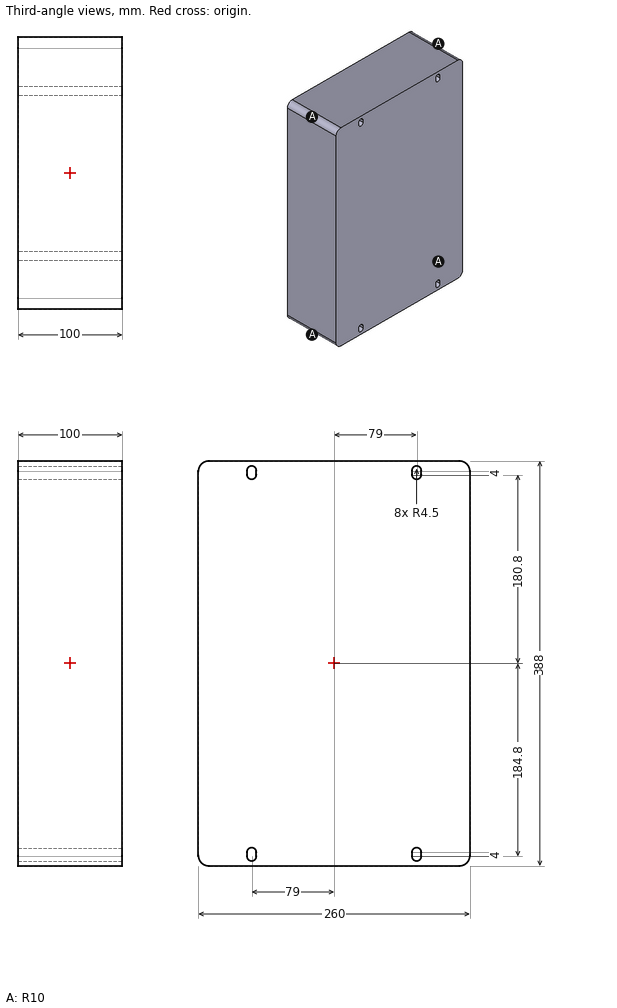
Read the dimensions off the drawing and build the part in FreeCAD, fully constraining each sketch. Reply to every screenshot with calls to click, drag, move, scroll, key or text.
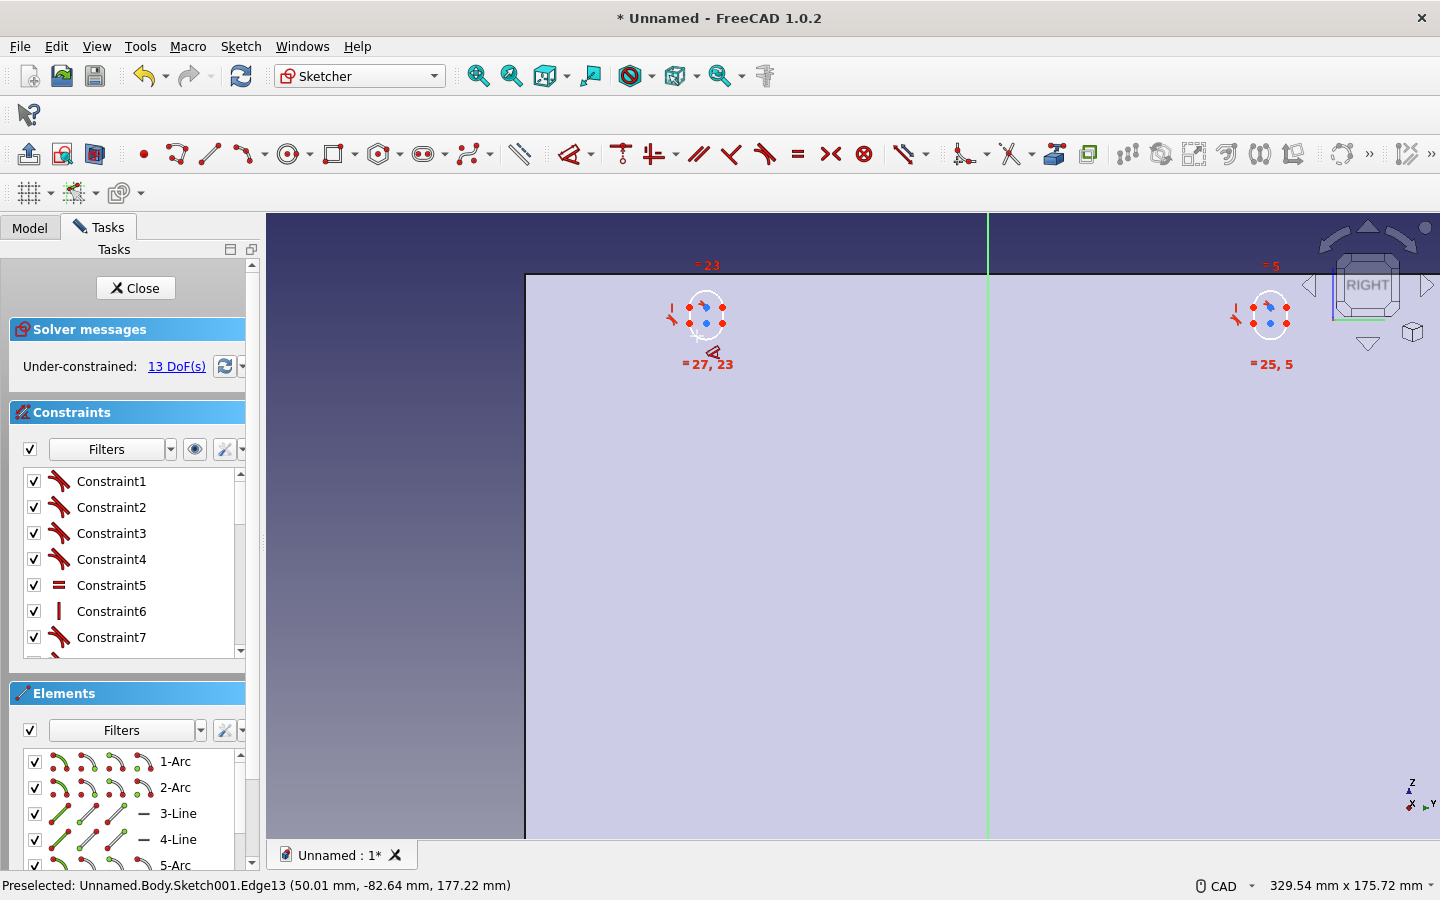
scroll(1261, 336, up, 5)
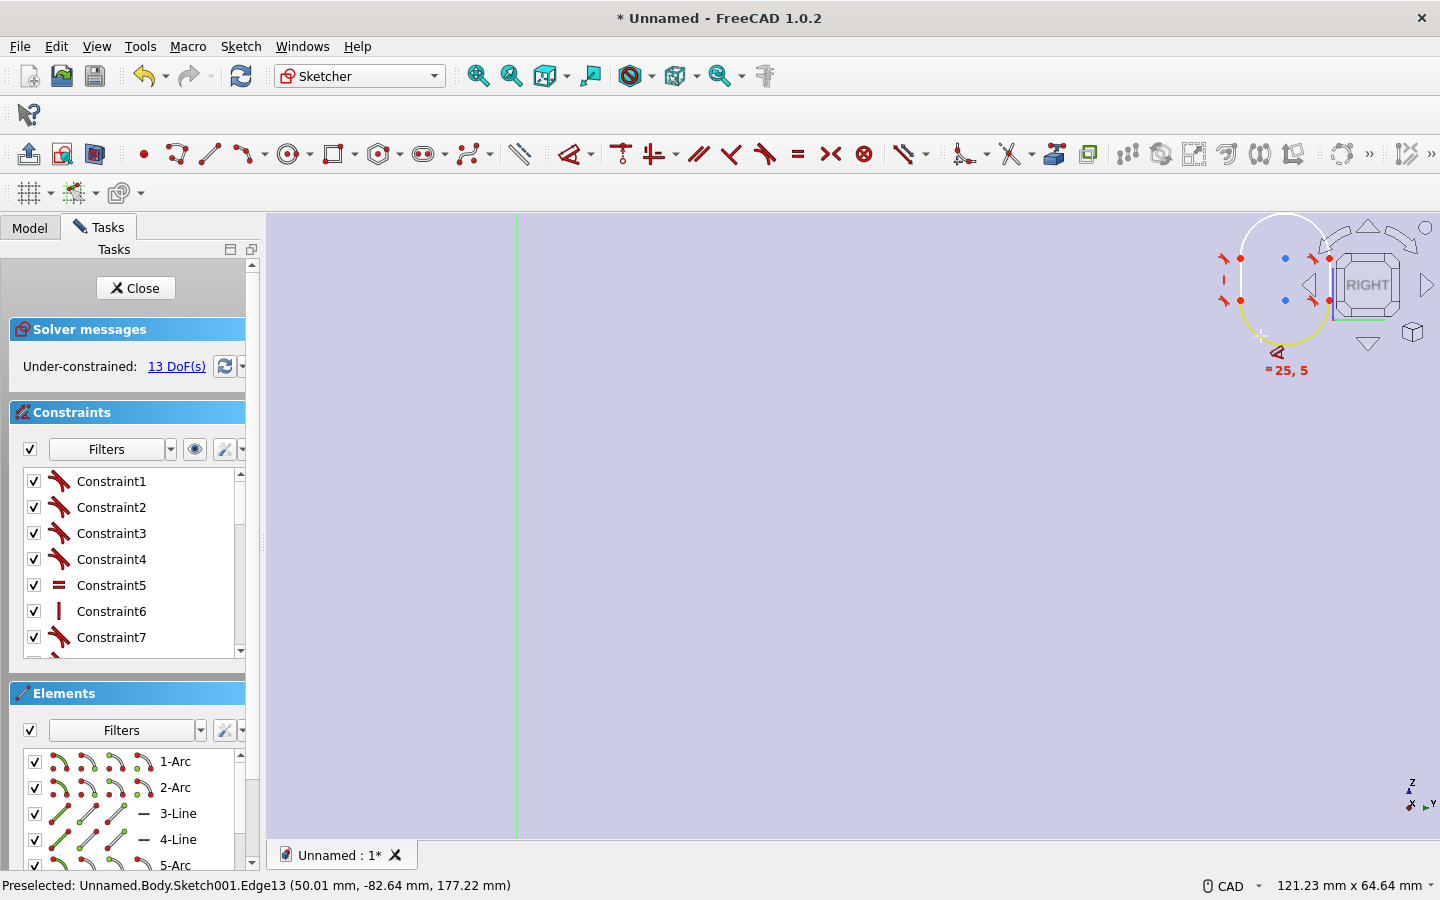
click(1259, 337)
click(1240, 363)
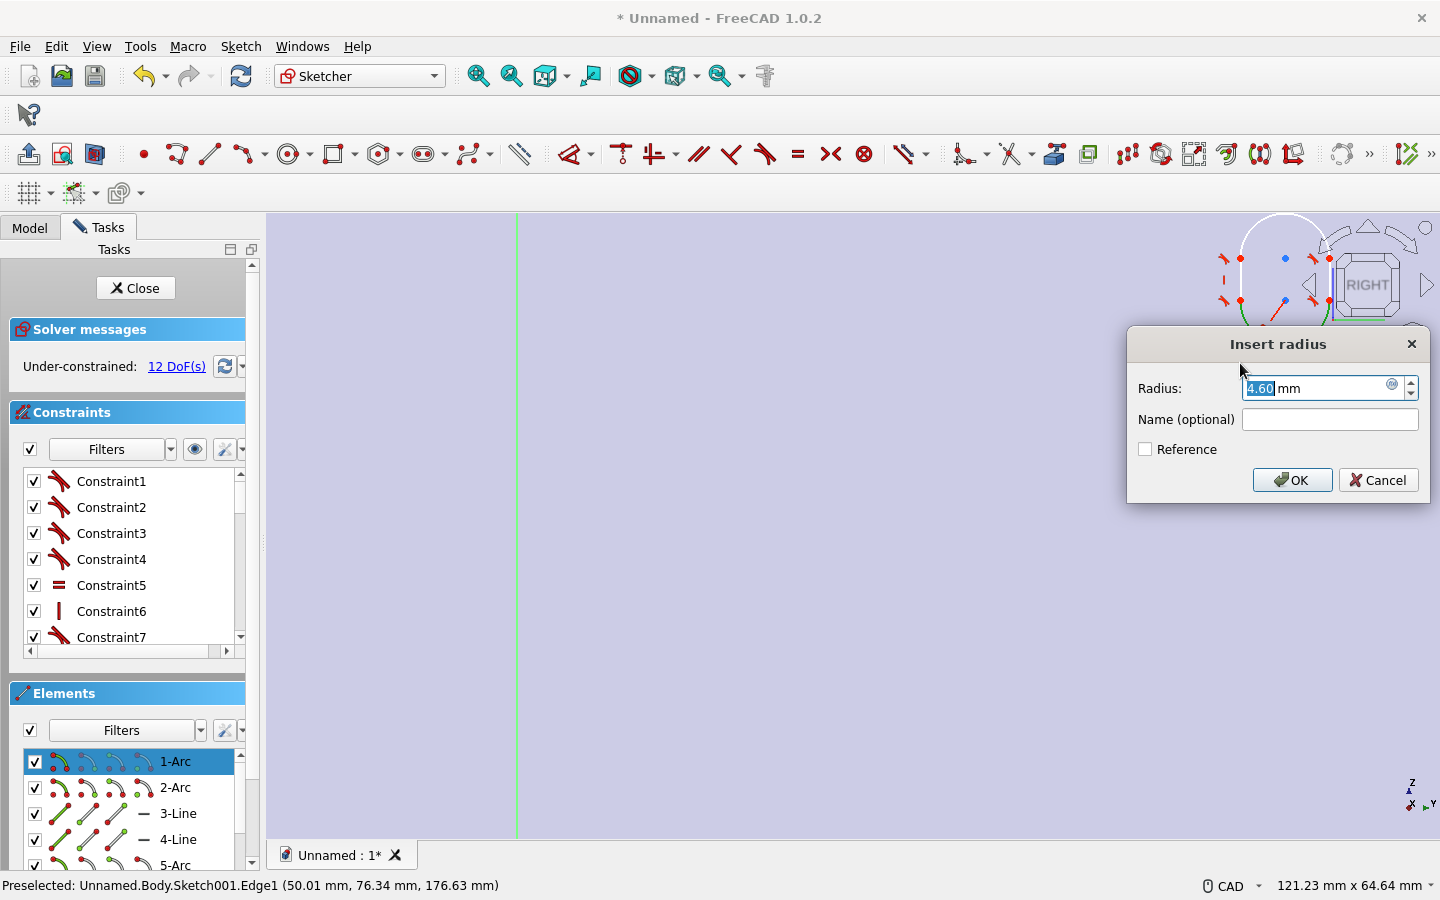
text(4.5)
key(Return)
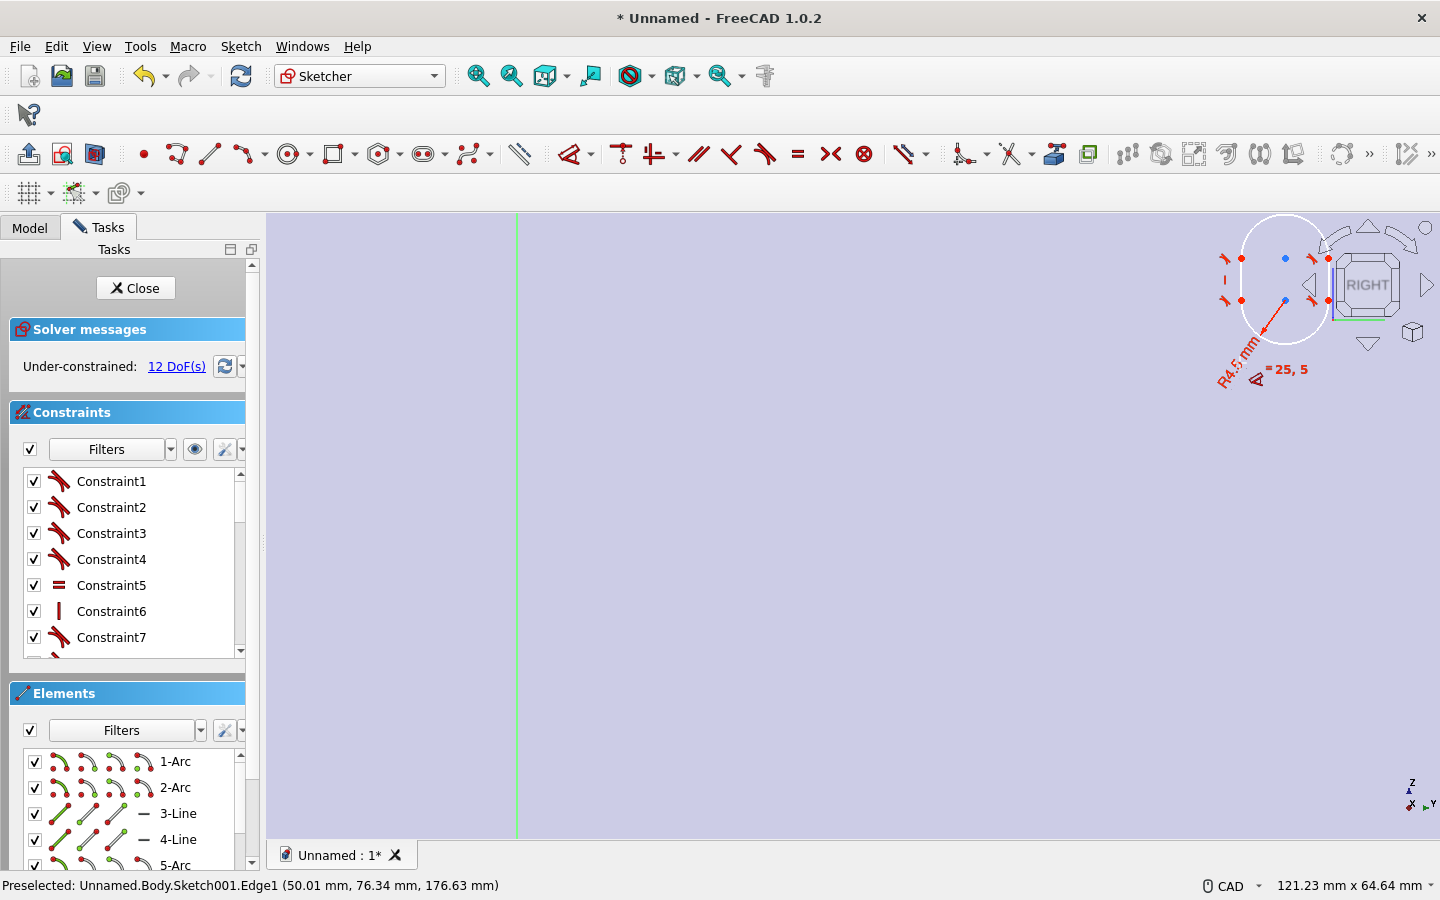
click(1241, 288)
click(1207, 279)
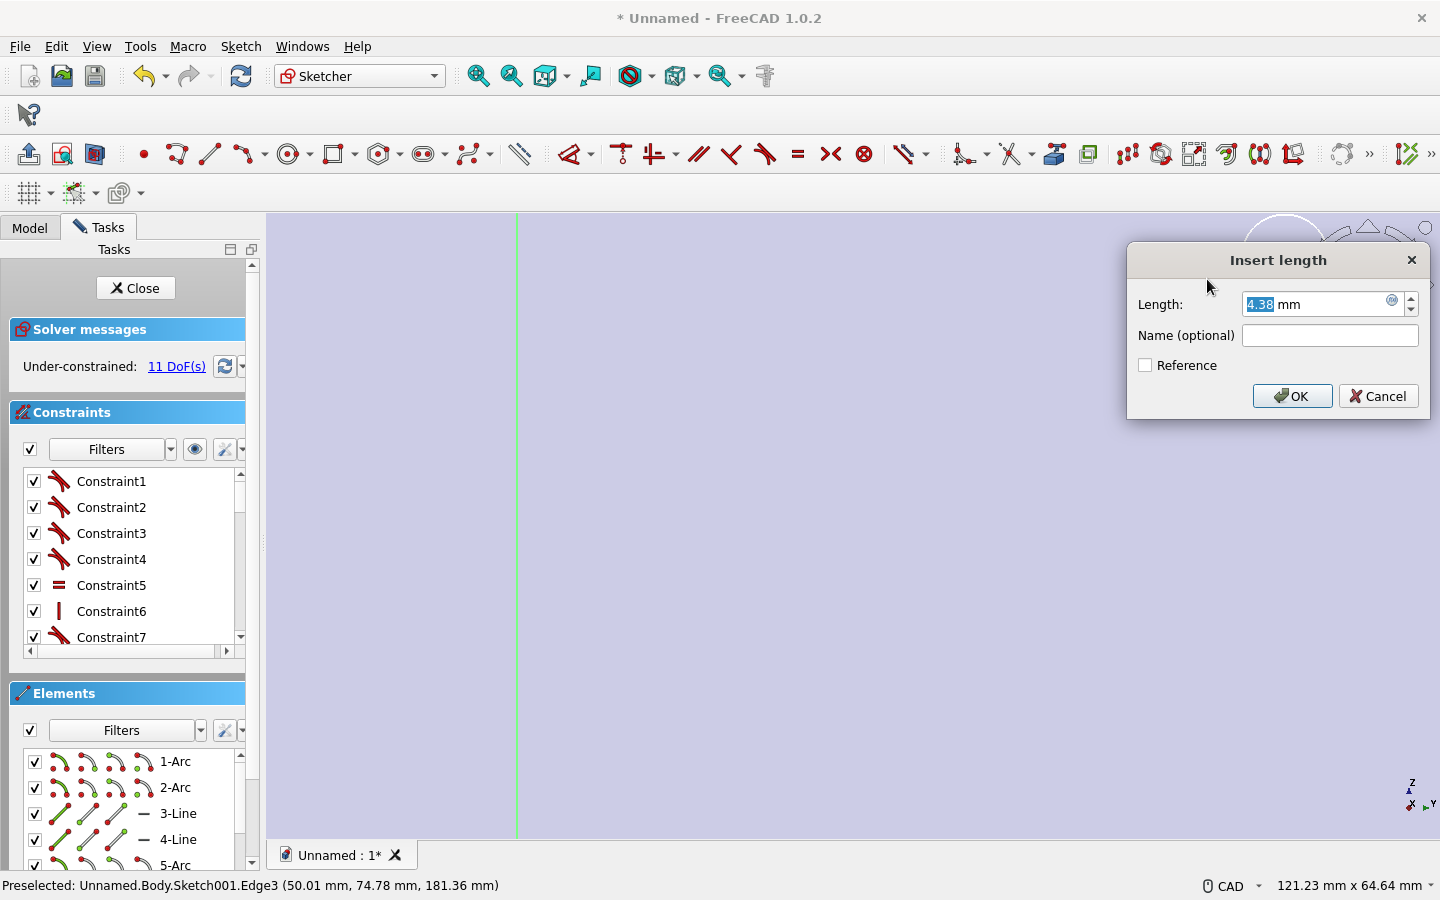
text(4)
key(Return)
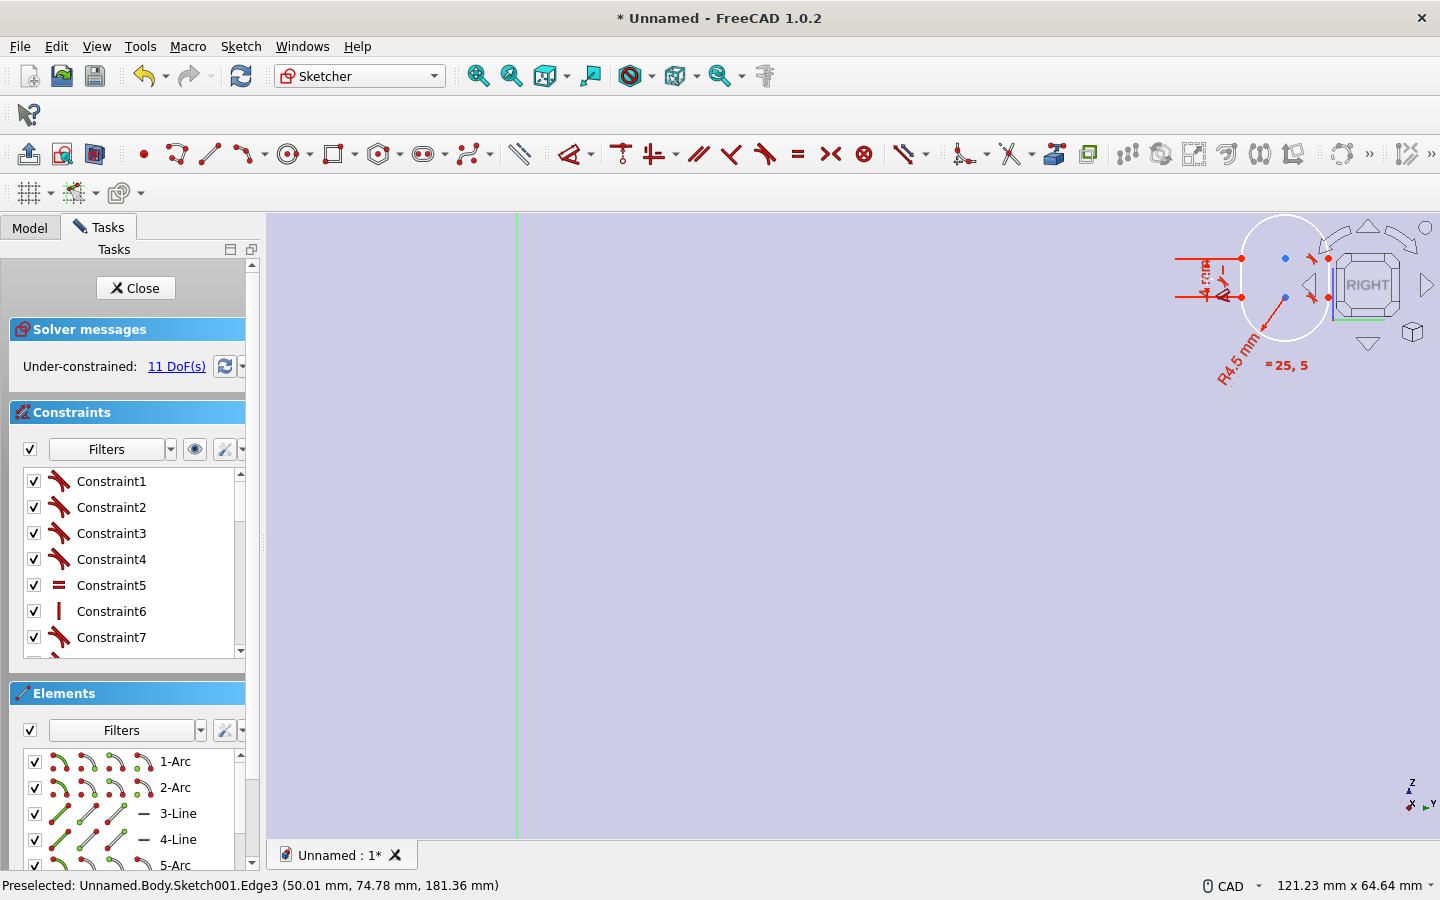
scroll(818, 337, down, 11)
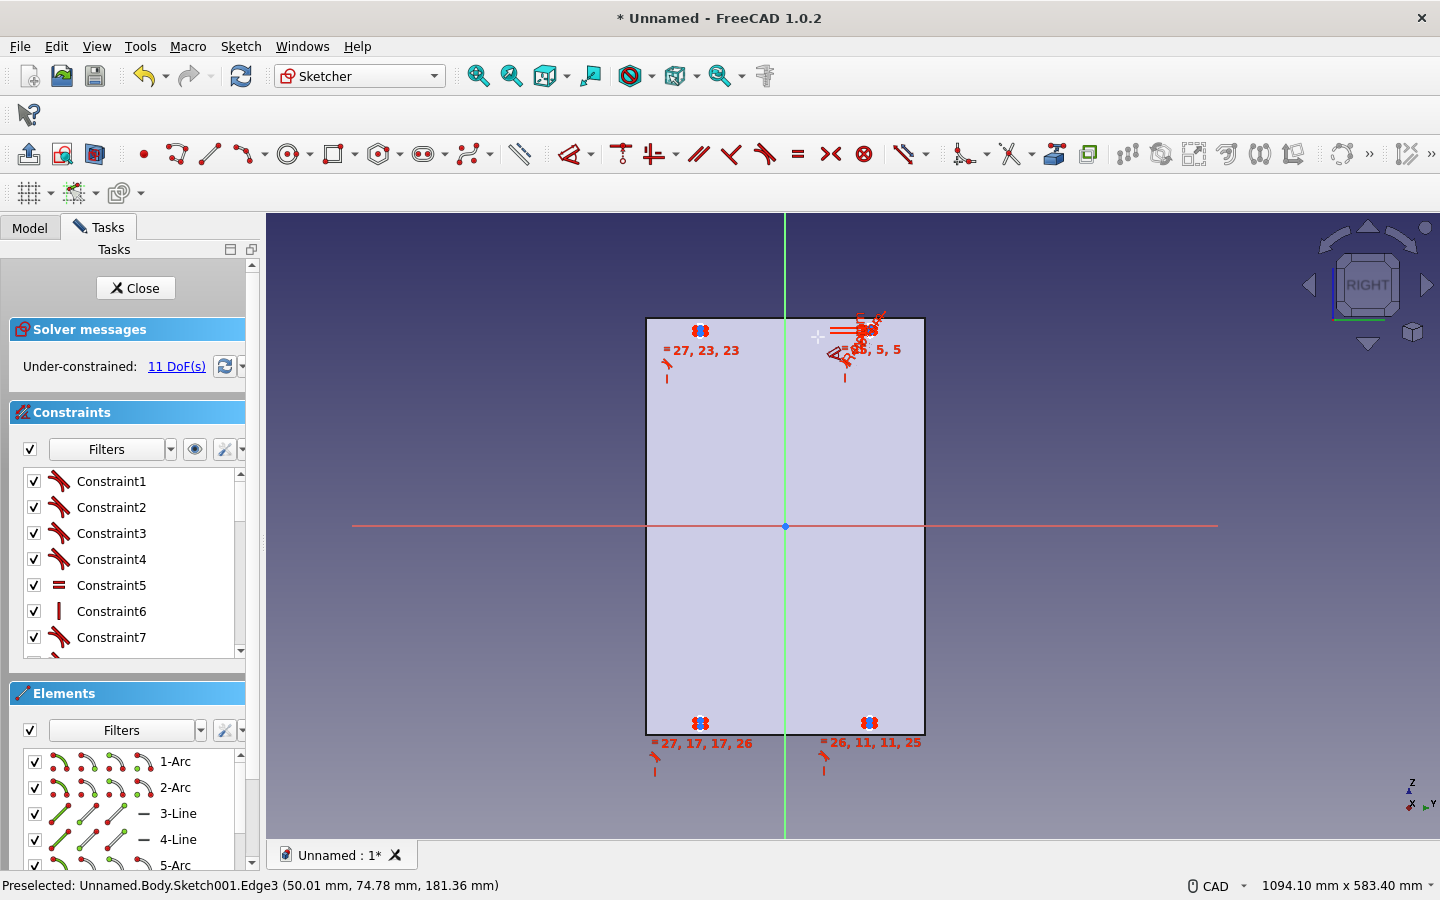
scroll(865, 724, up, 12)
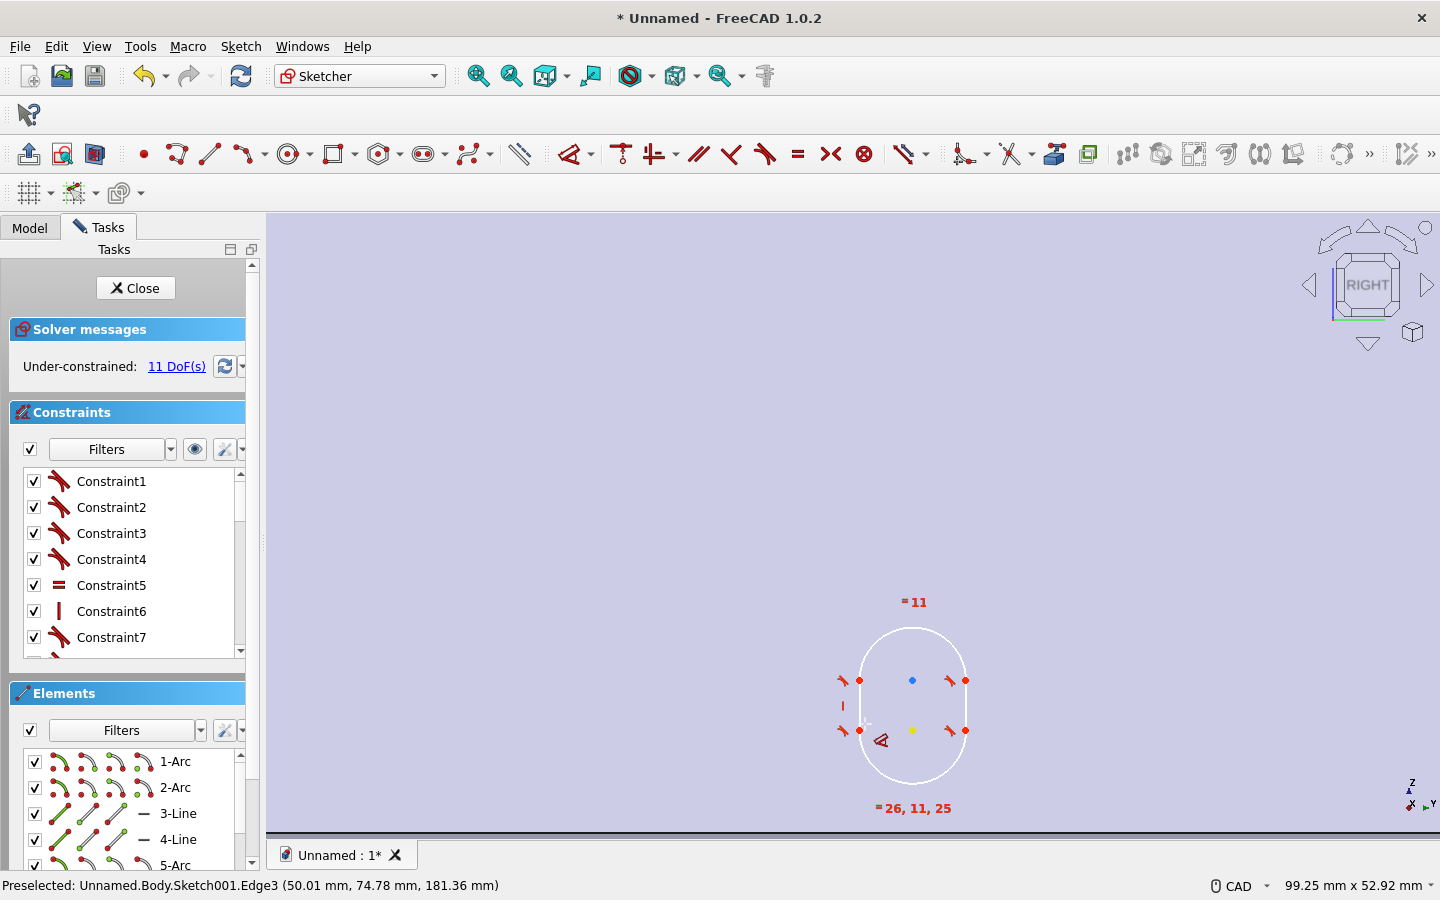
click(860, 716)
click(894, 706)